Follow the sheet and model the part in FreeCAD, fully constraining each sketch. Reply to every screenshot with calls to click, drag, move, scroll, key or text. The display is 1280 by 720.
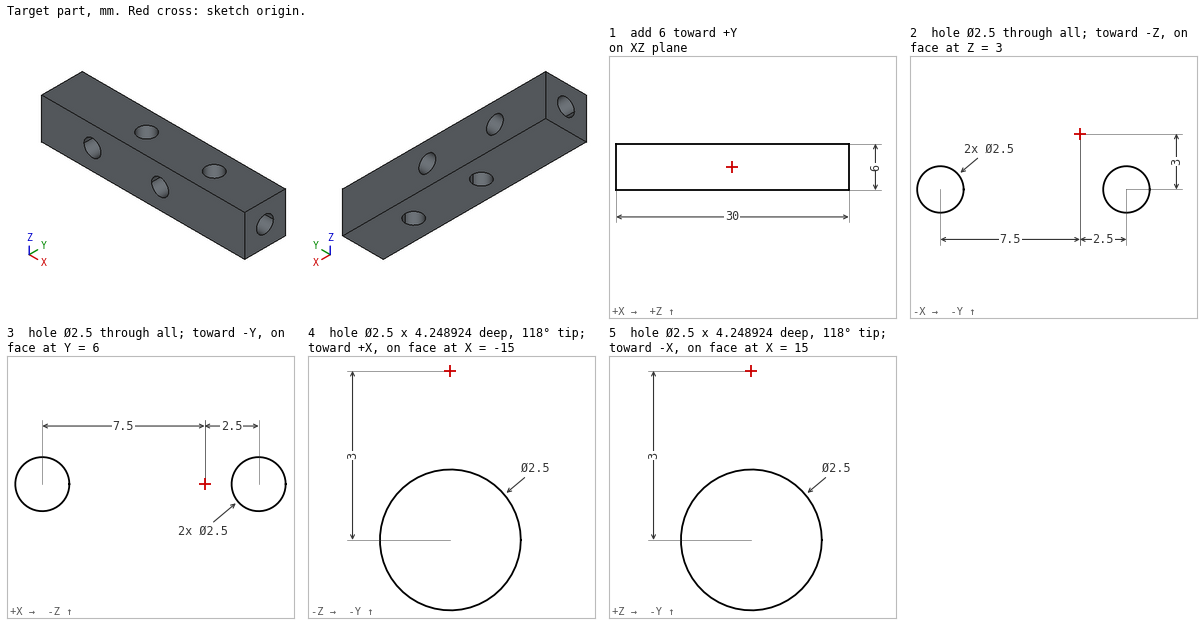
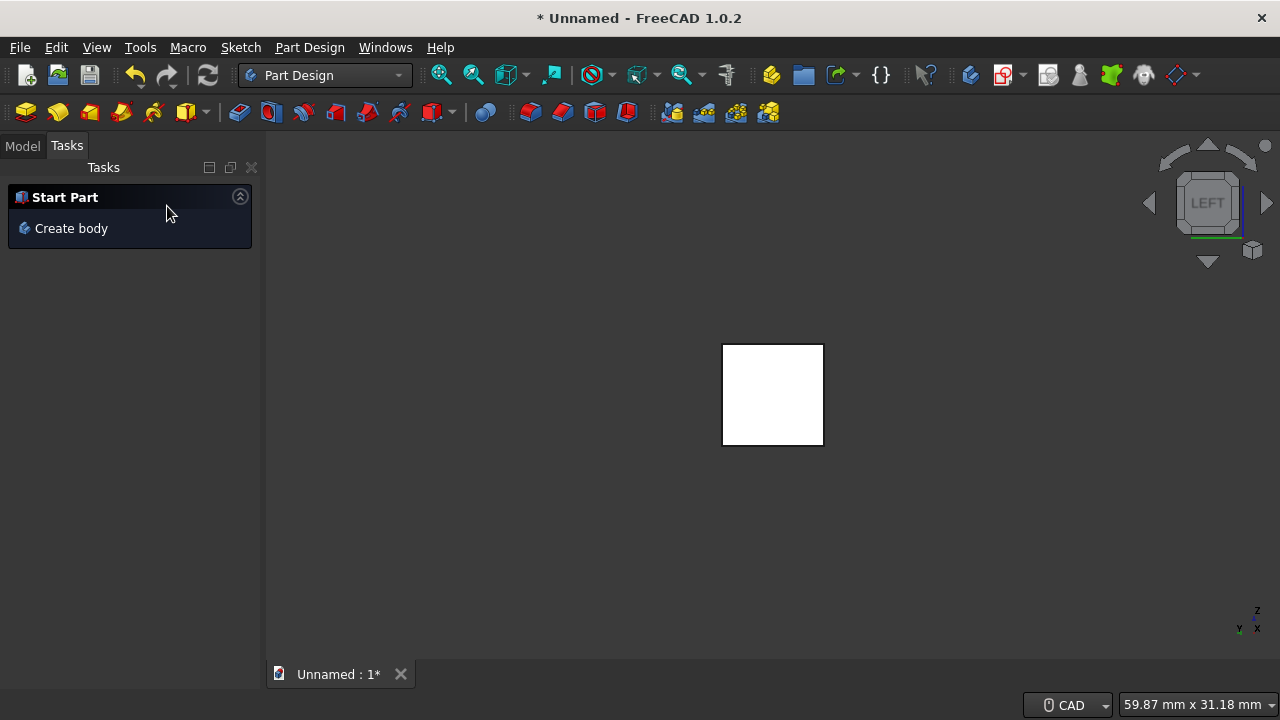
click(773, 394)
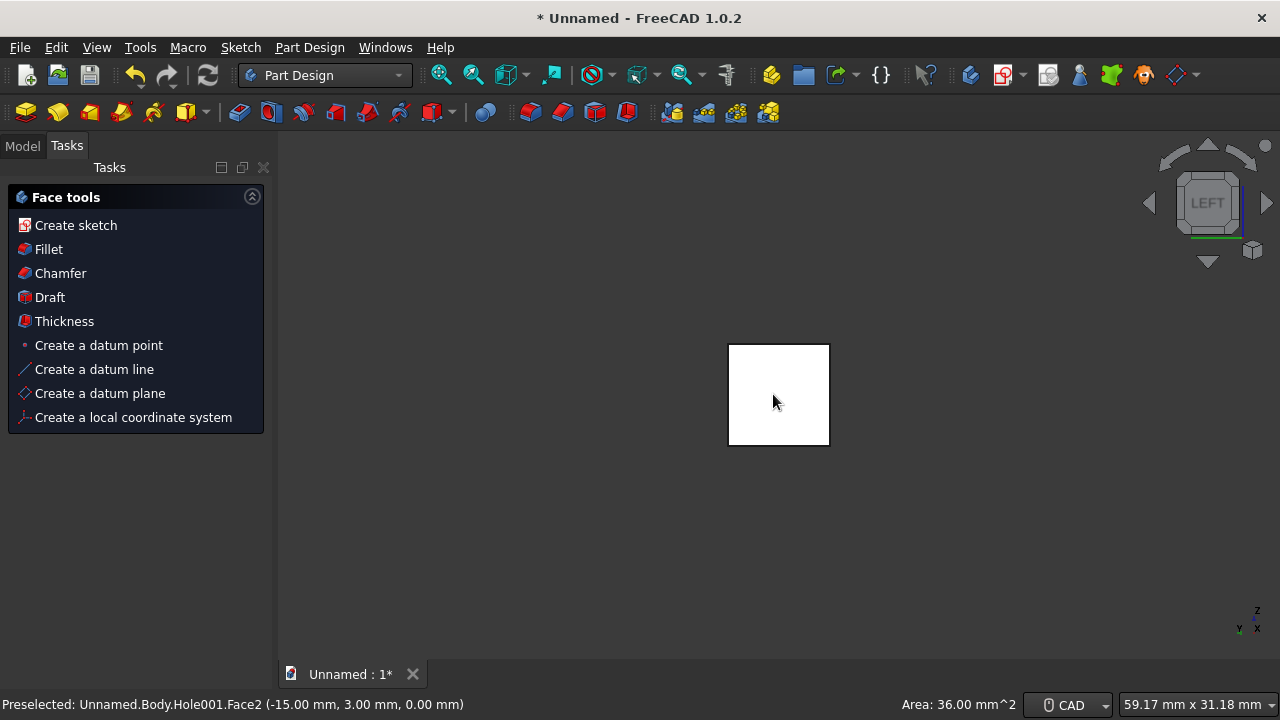
click(1004, 76)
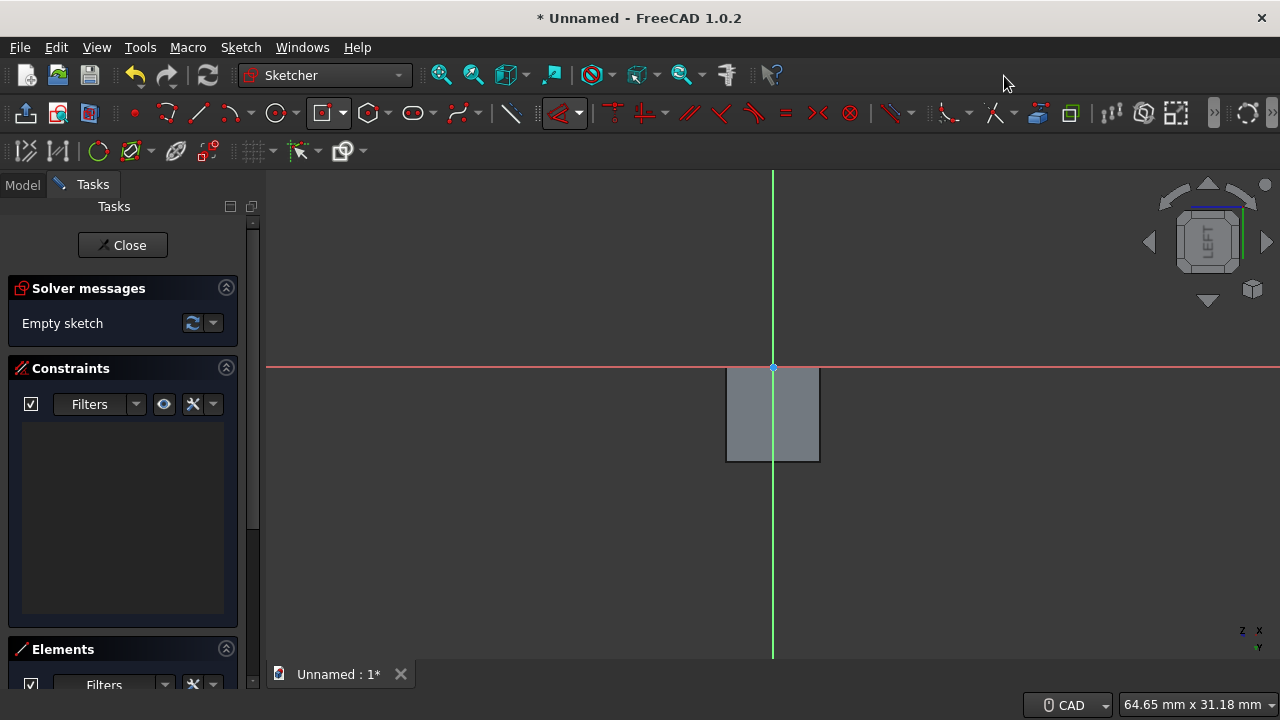
scroll(790, 397, up, 8)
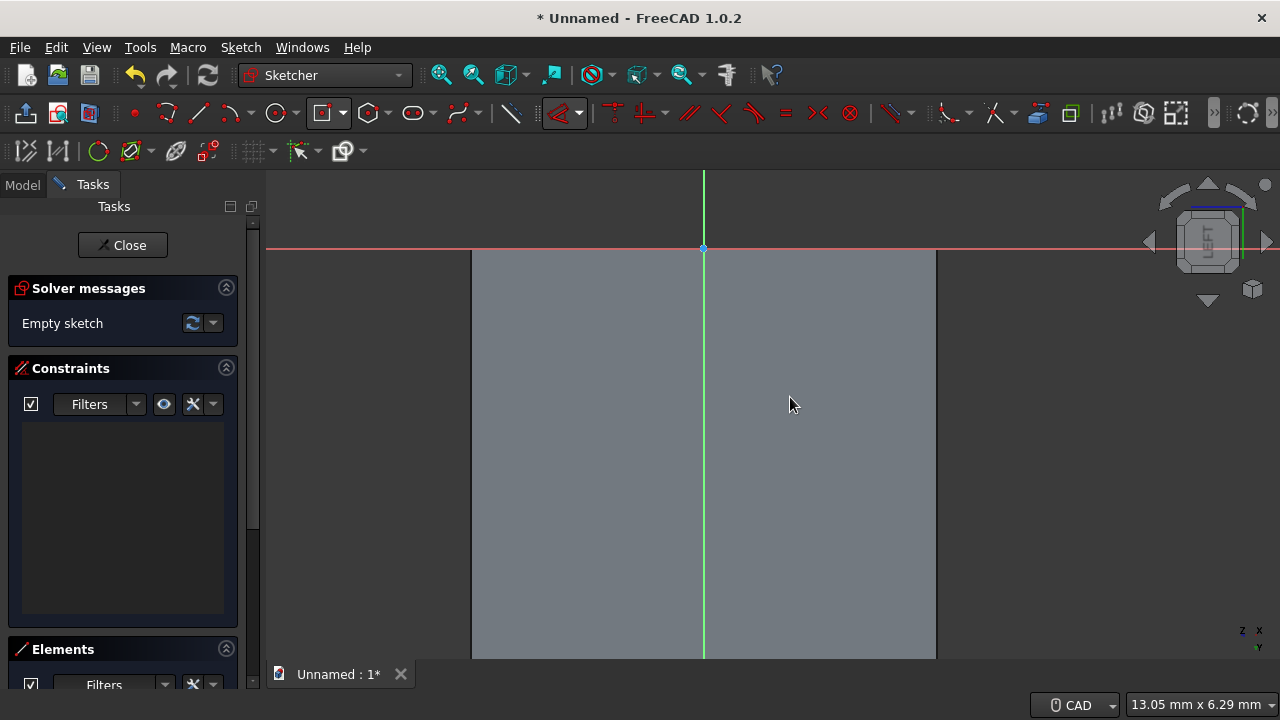
click(276, 114)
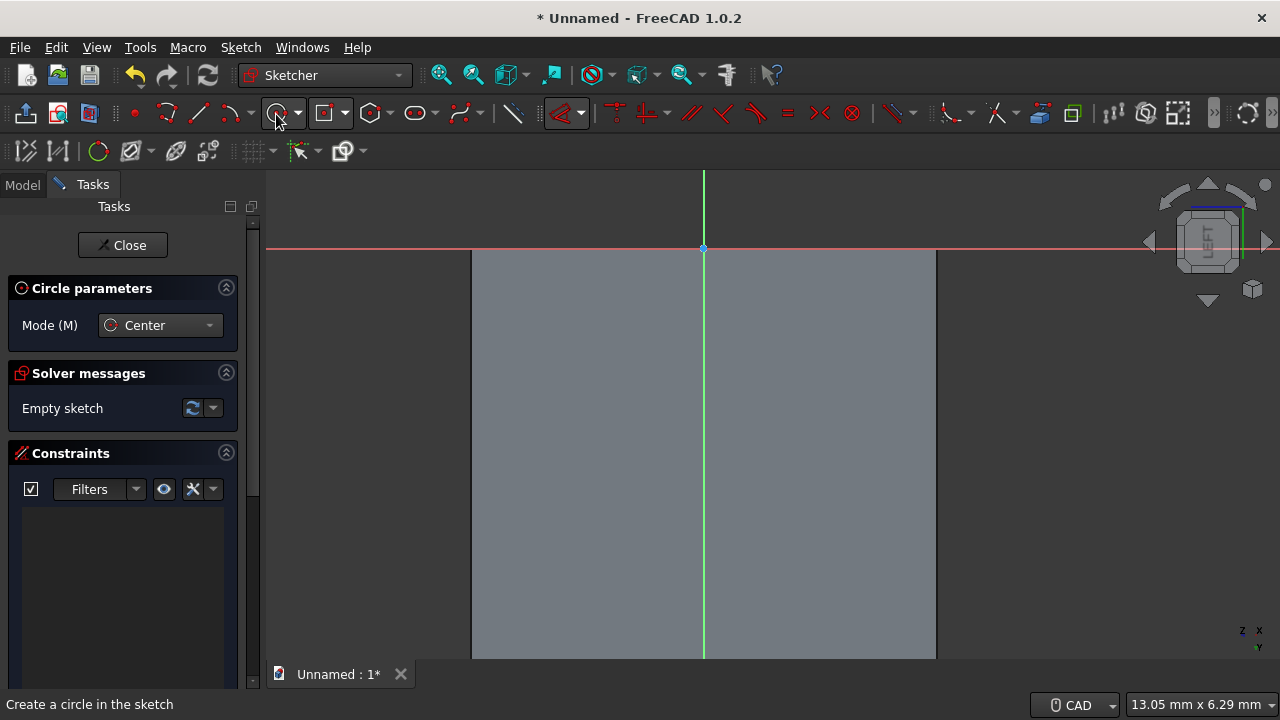
click(704, 482)
move(772, 413)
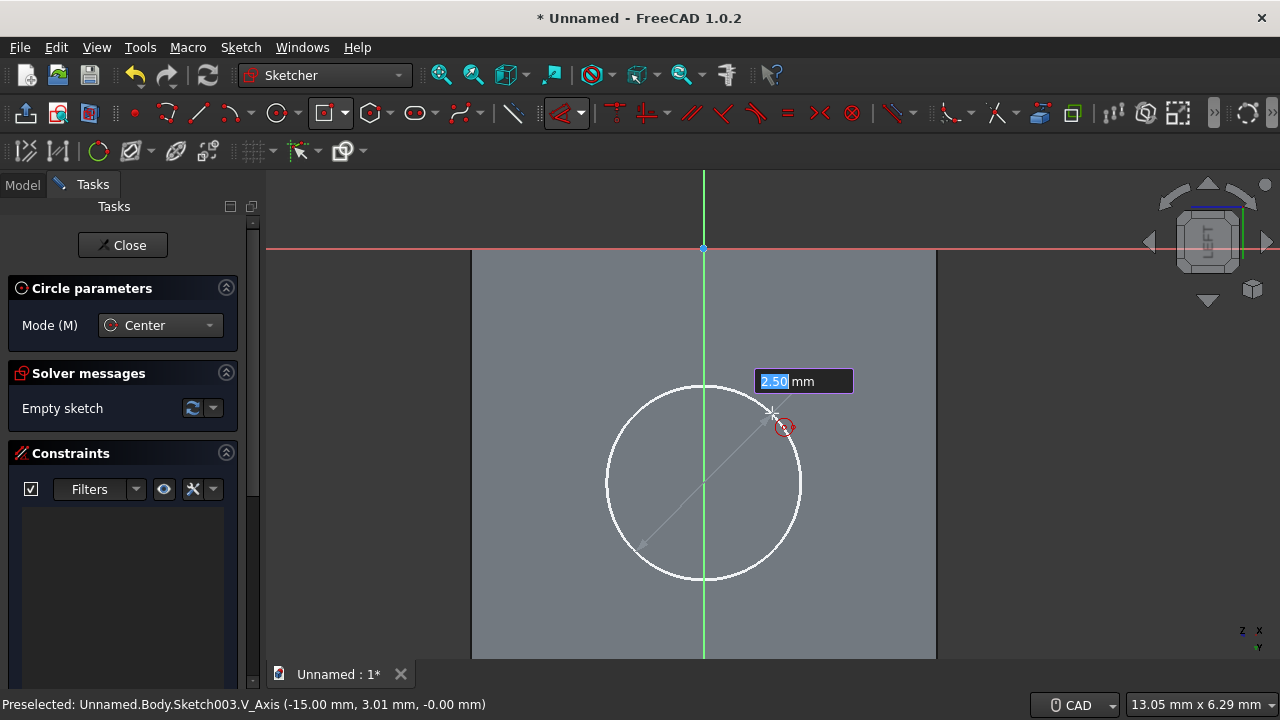
text(2.5)
key(Return)
key(Escape)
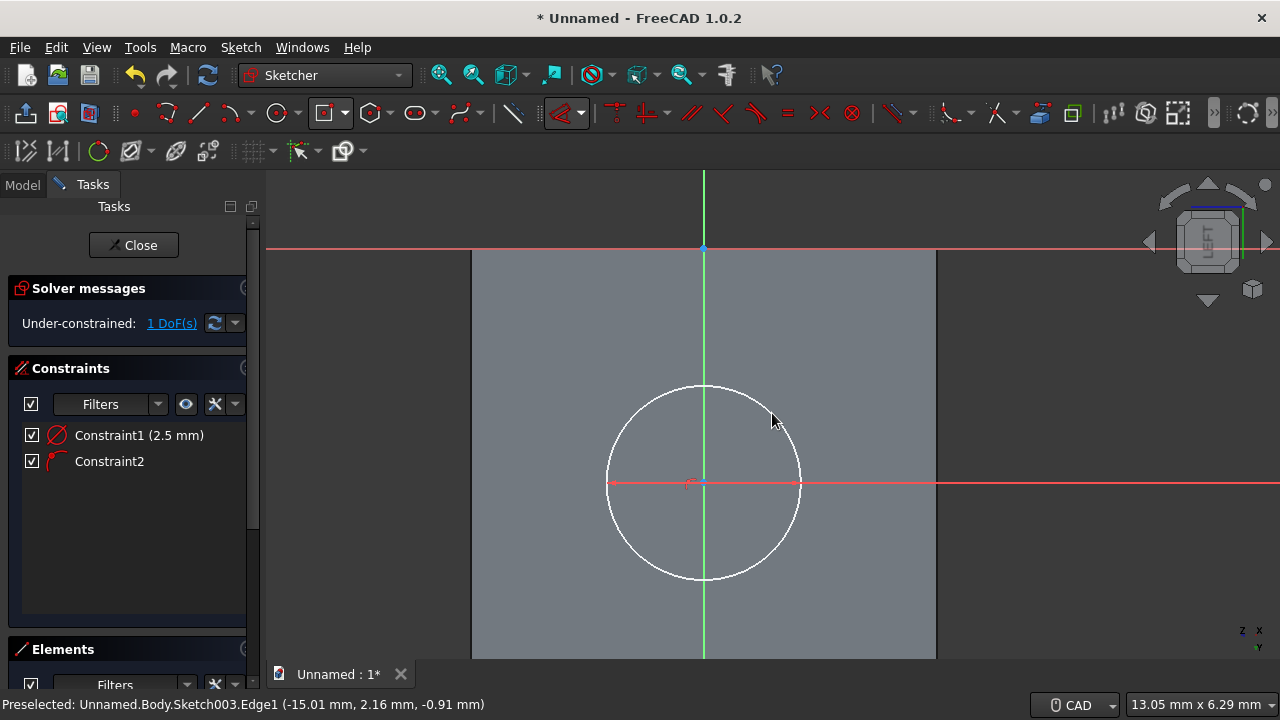
click(706, 485)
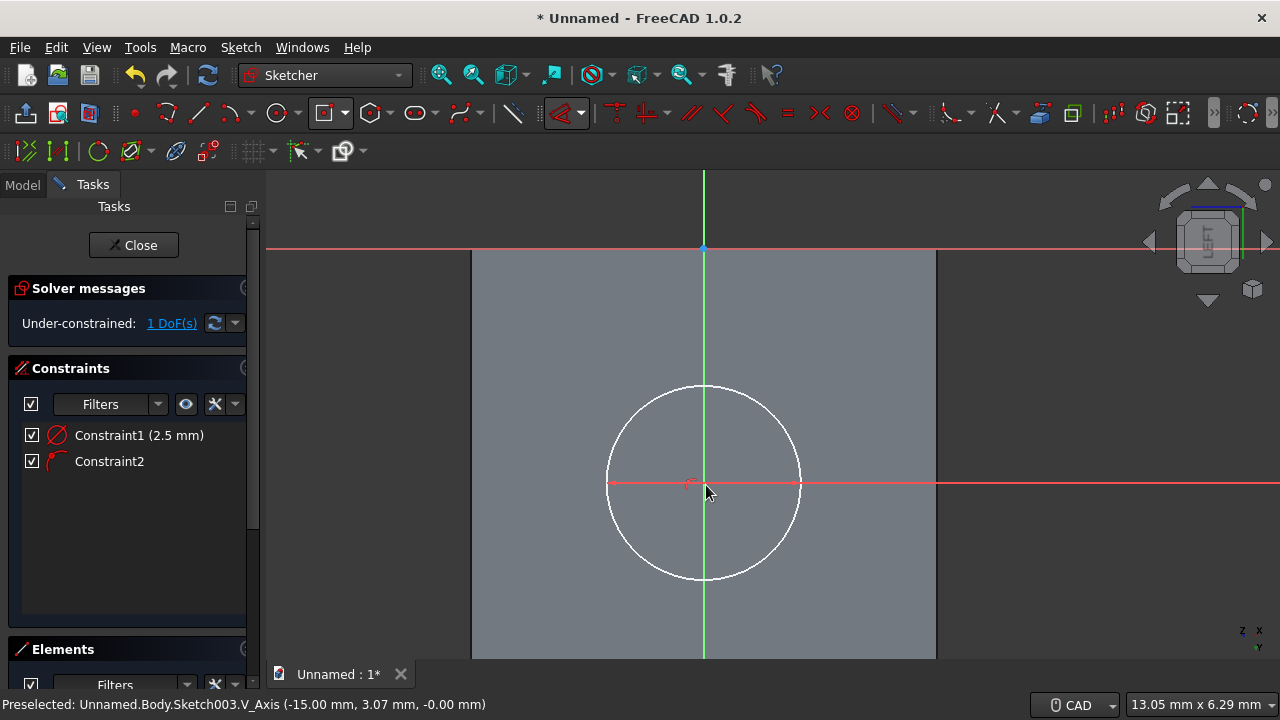
key(i)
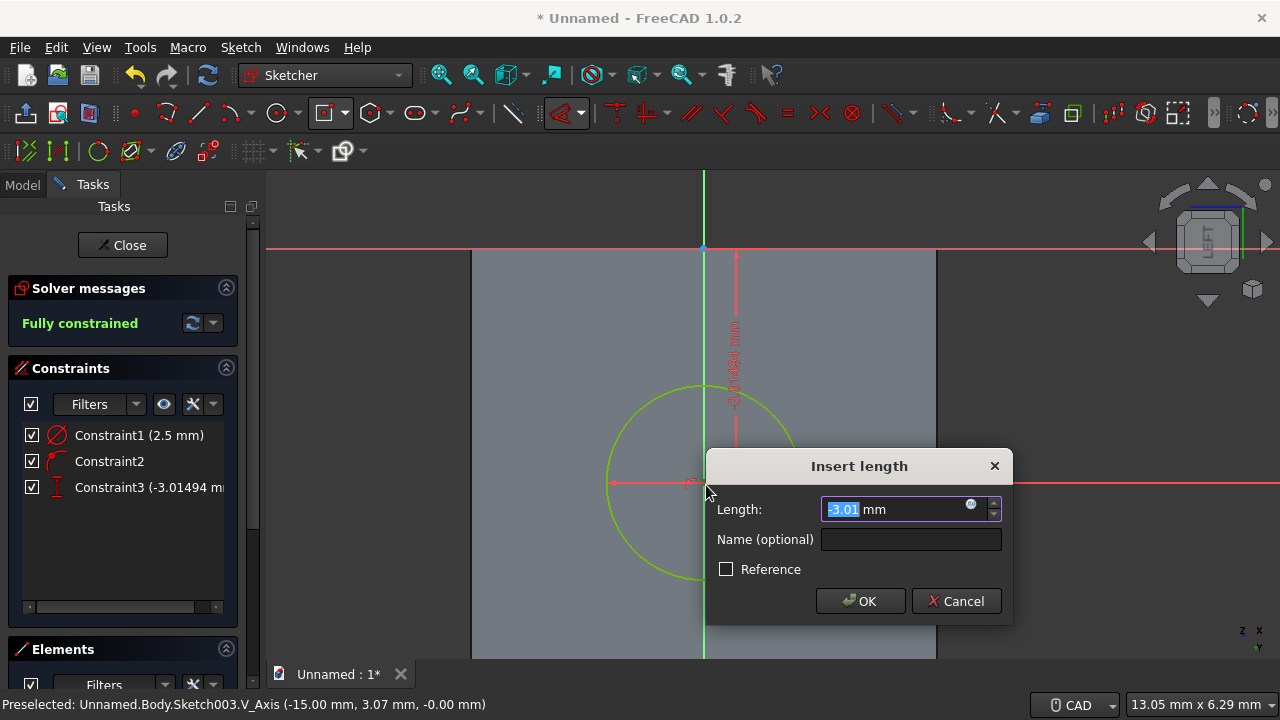
text(-3)
key(Return)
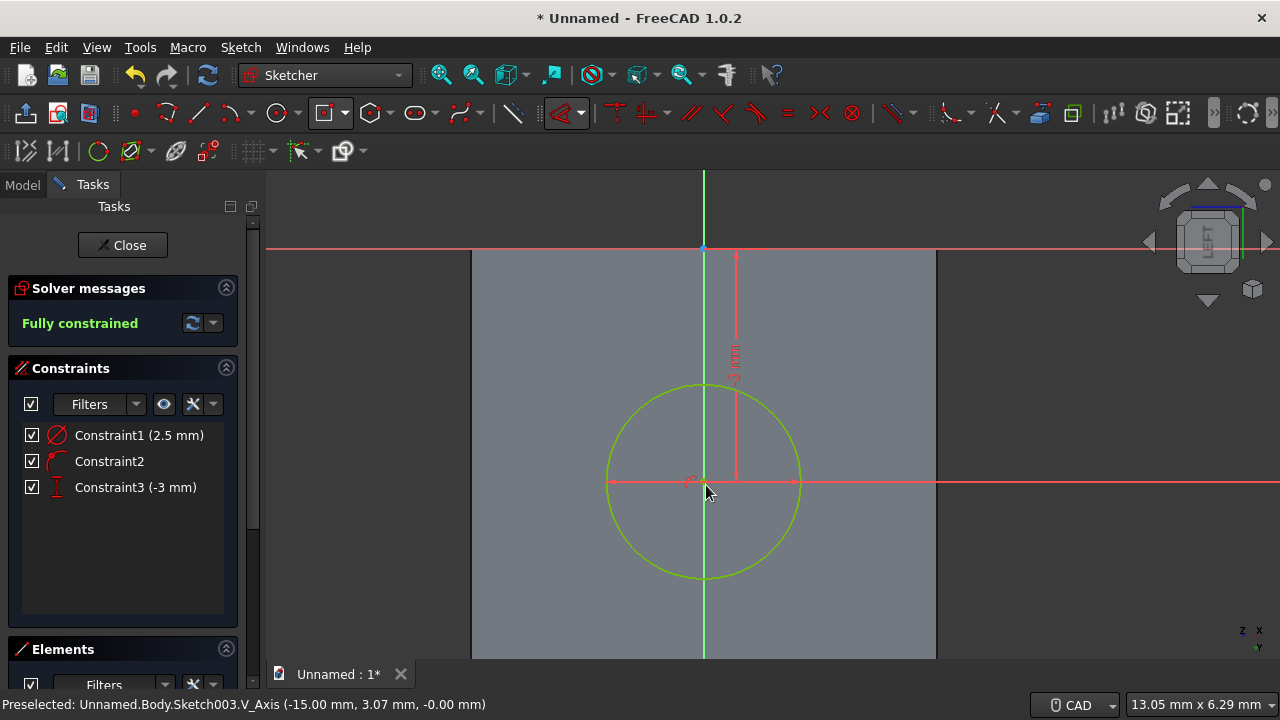
click(123, 245)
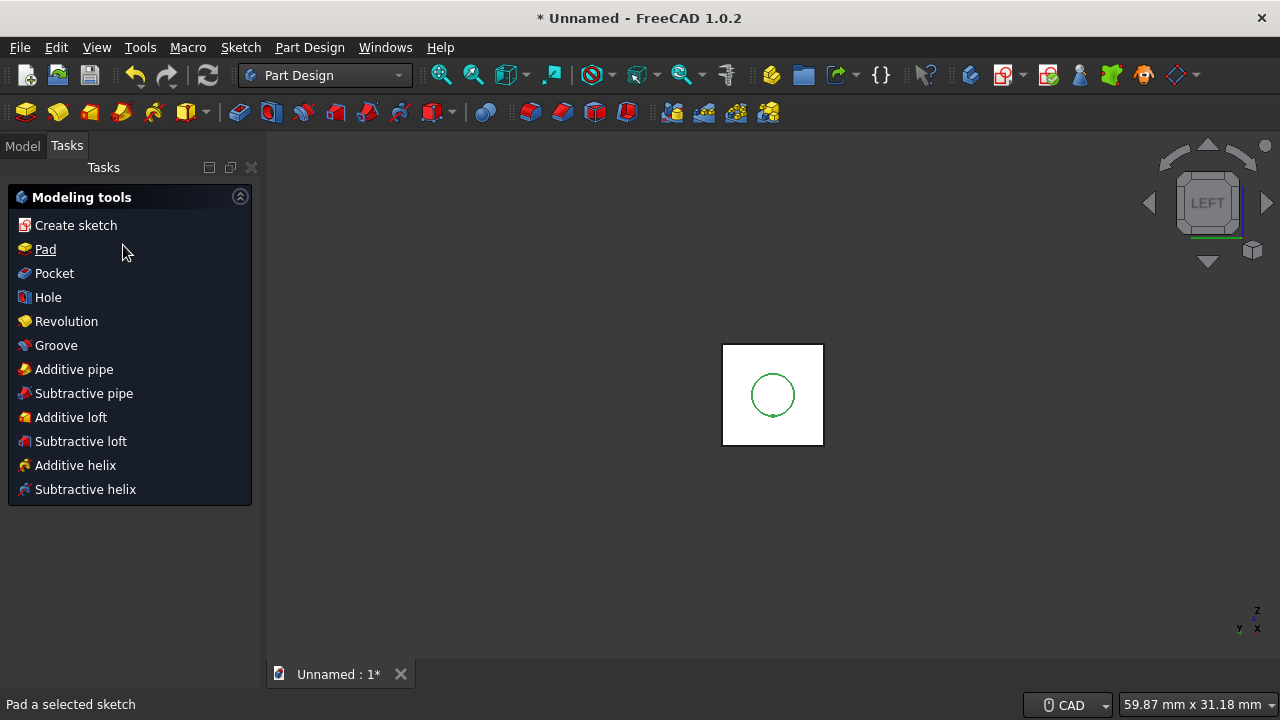
click(272, 112)